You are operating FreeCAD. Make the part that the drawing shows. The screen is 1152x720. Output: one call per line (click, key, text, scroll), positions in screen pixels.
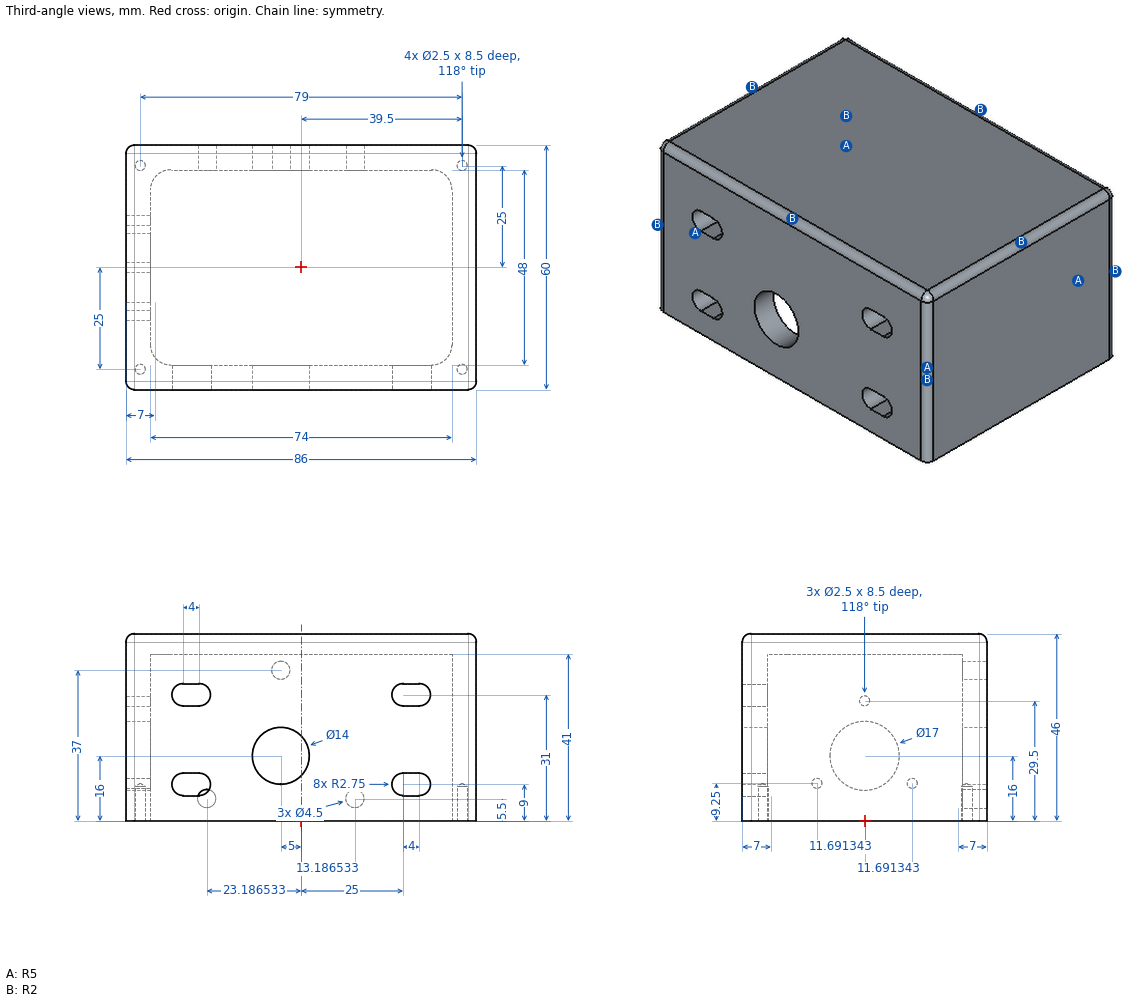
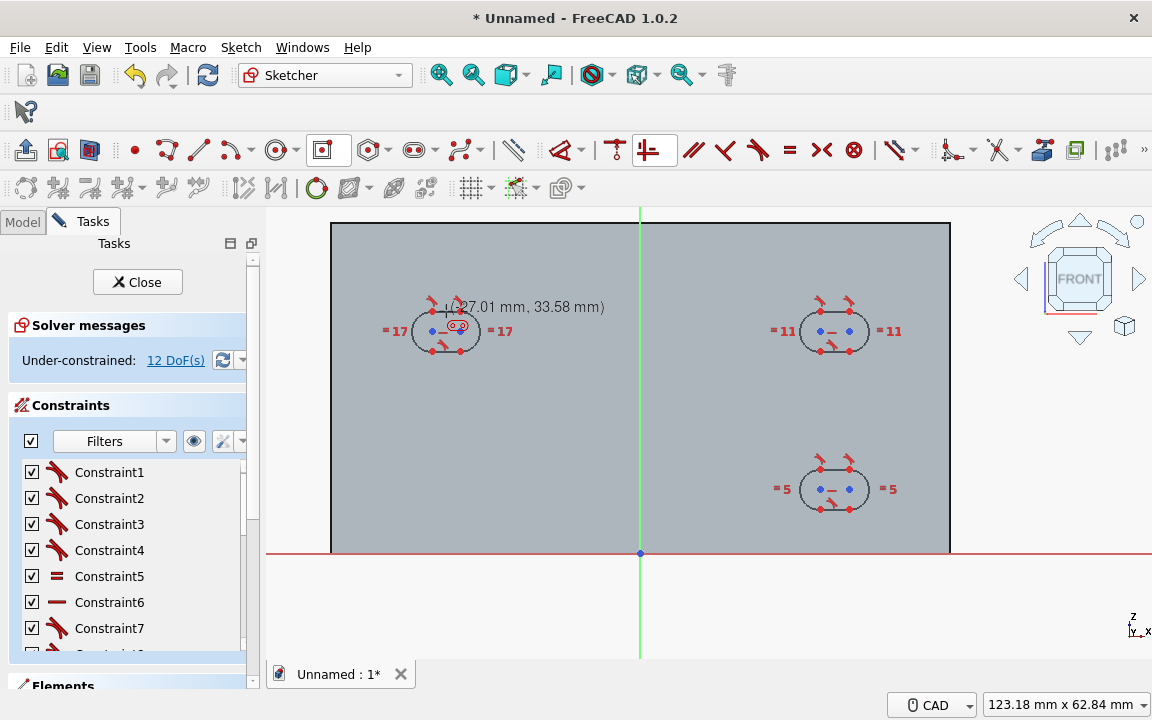
click(432, 489)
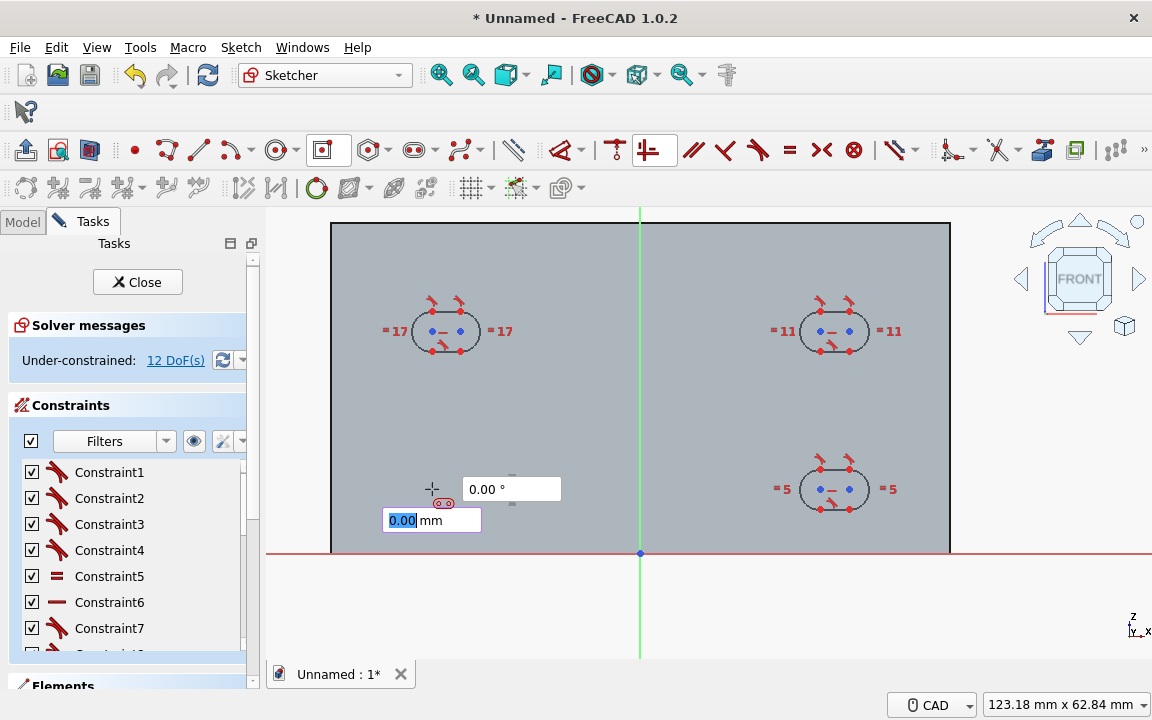
click(460, 489)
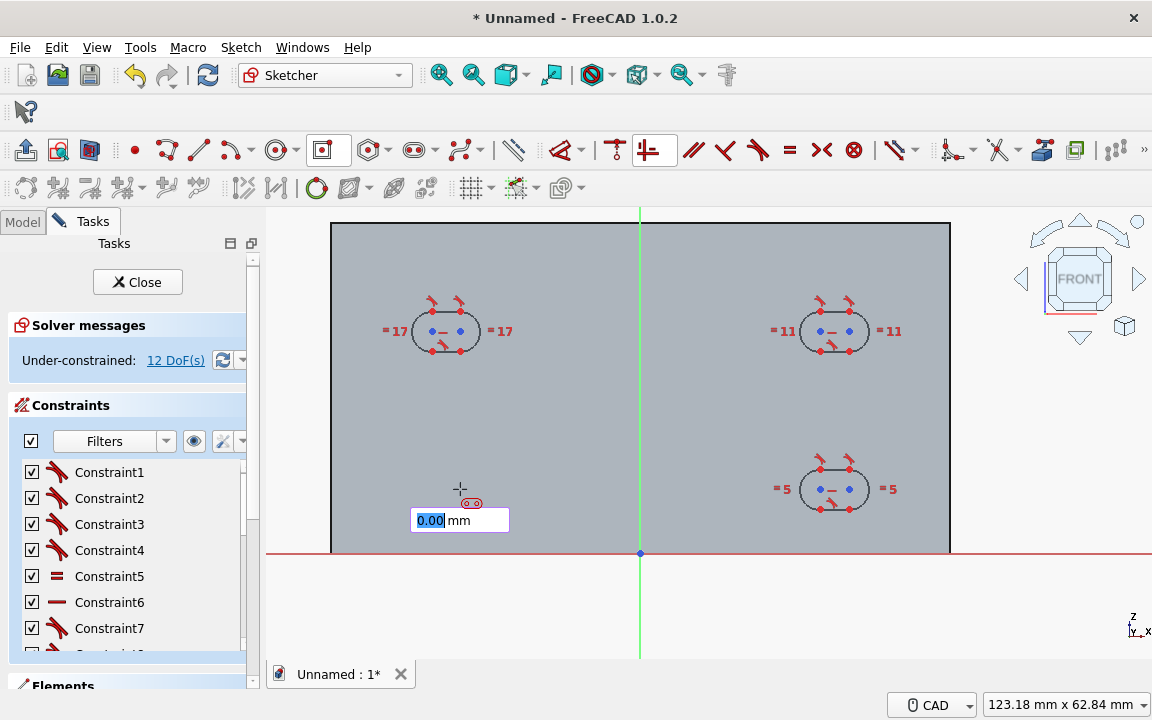
click(446, 469)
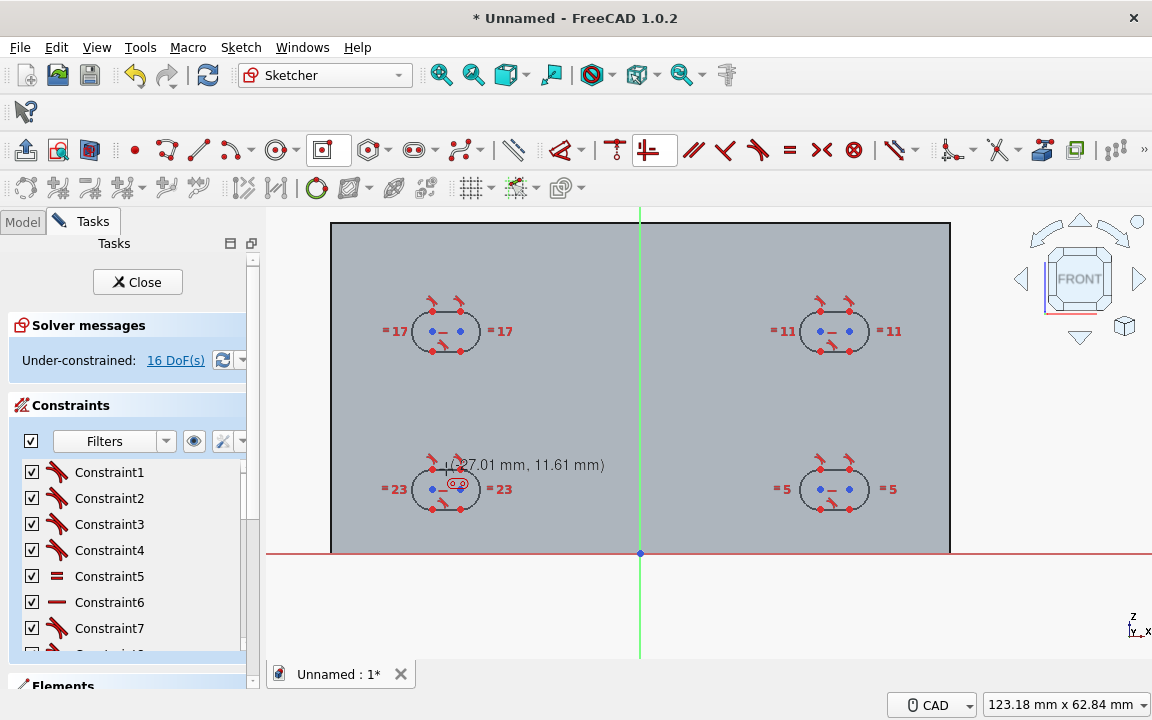
click(276, 150)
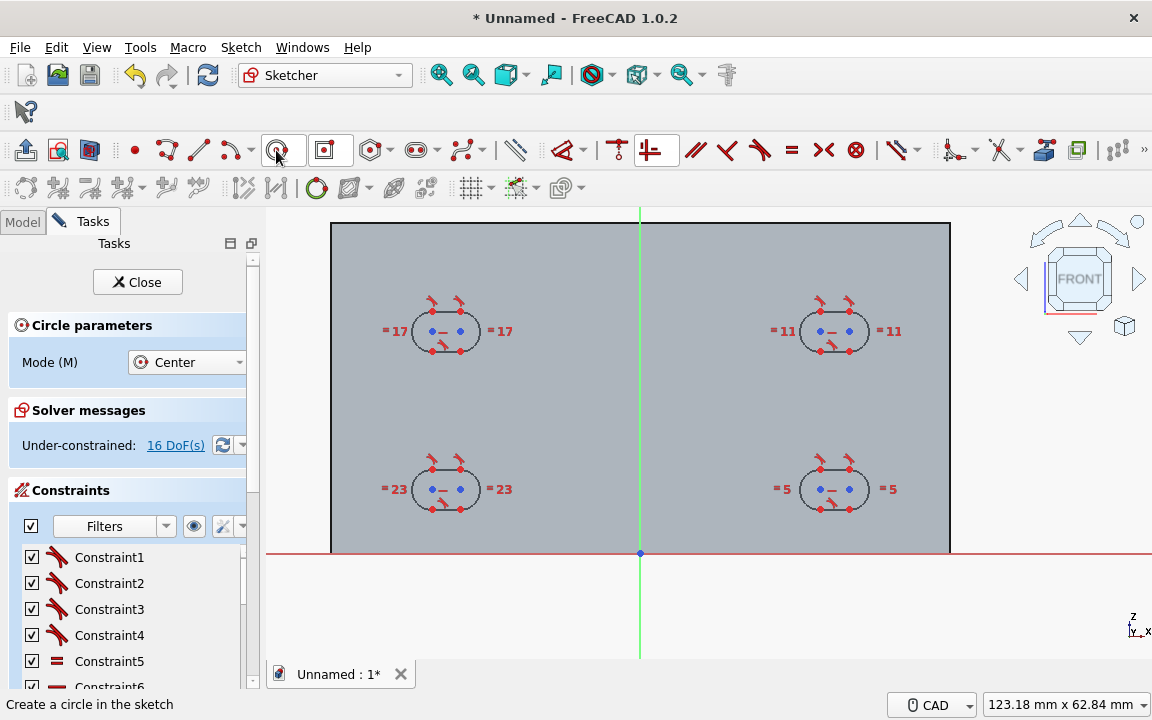
click(604, 438)
click(569, 403)
key(Escape)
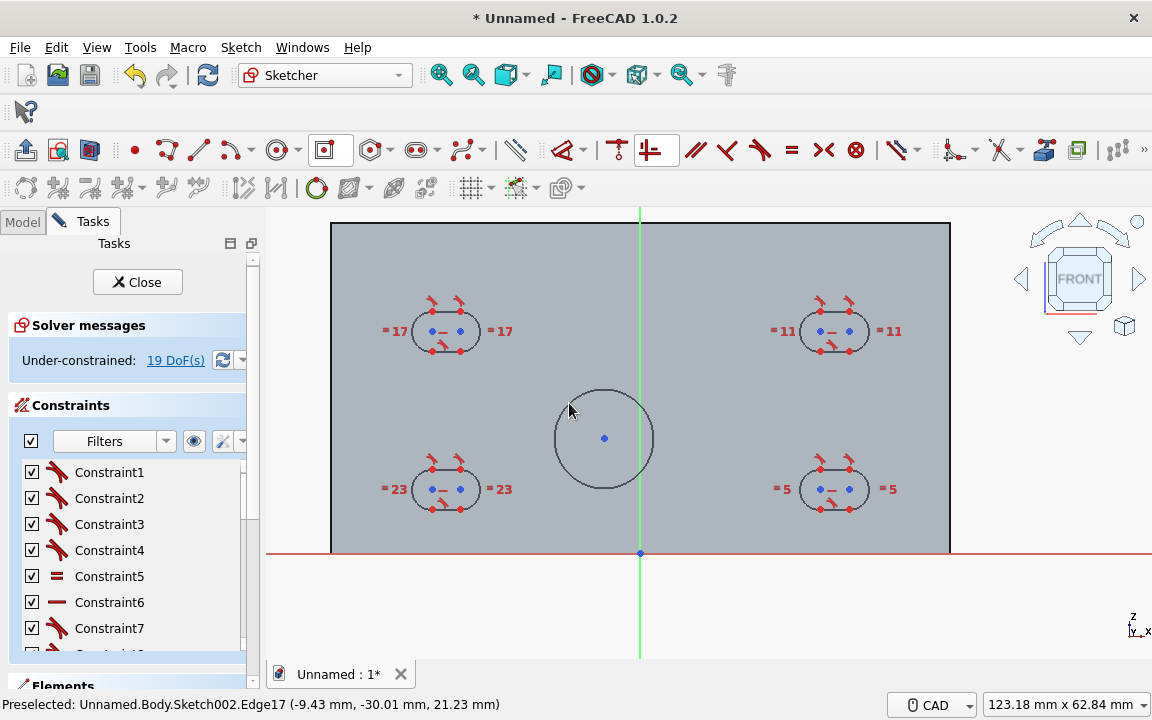
click(804, 478)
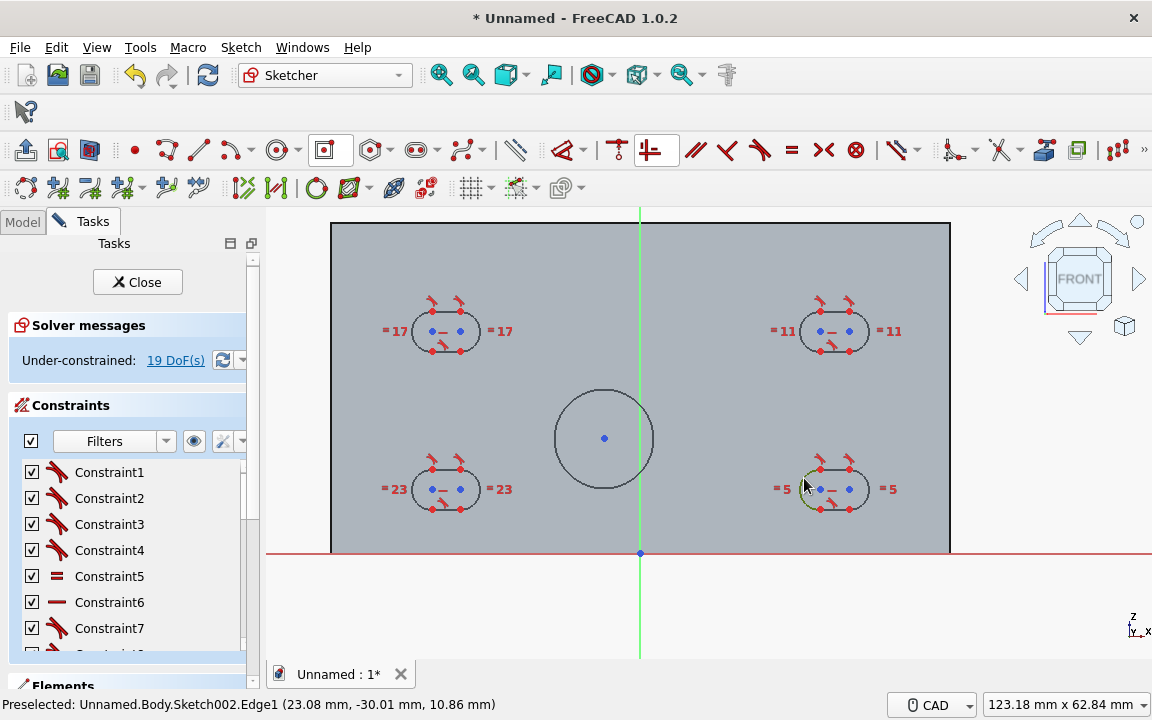
click(804, 320)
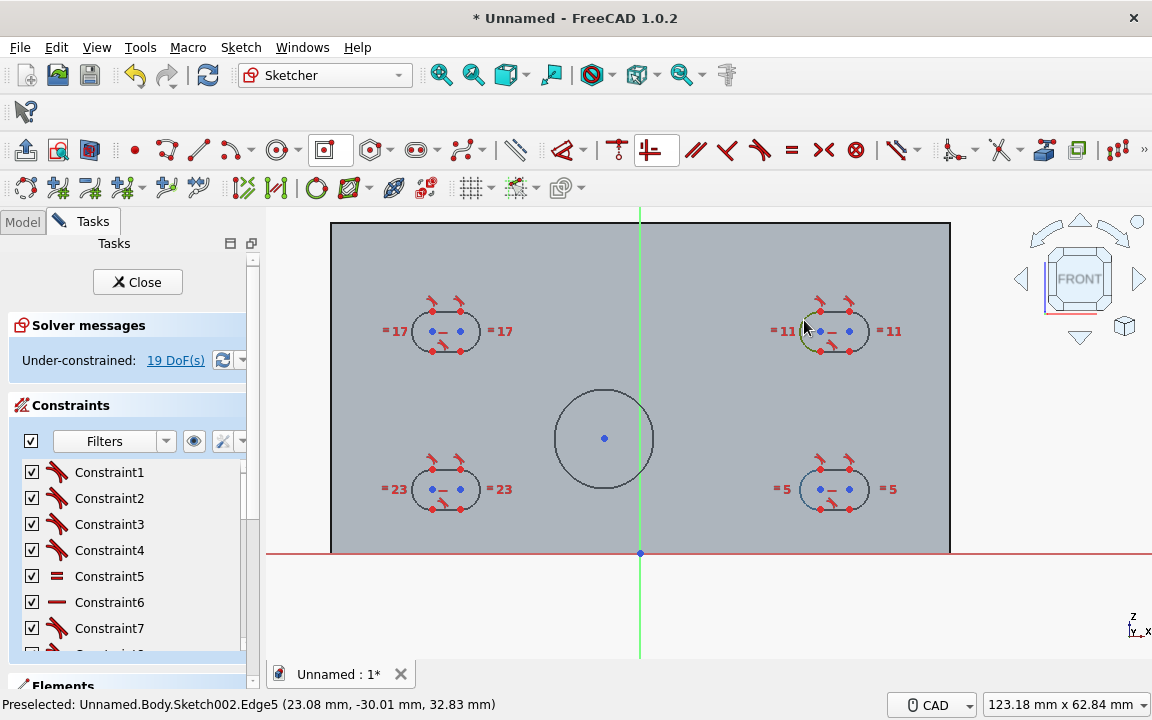
click(416, 320)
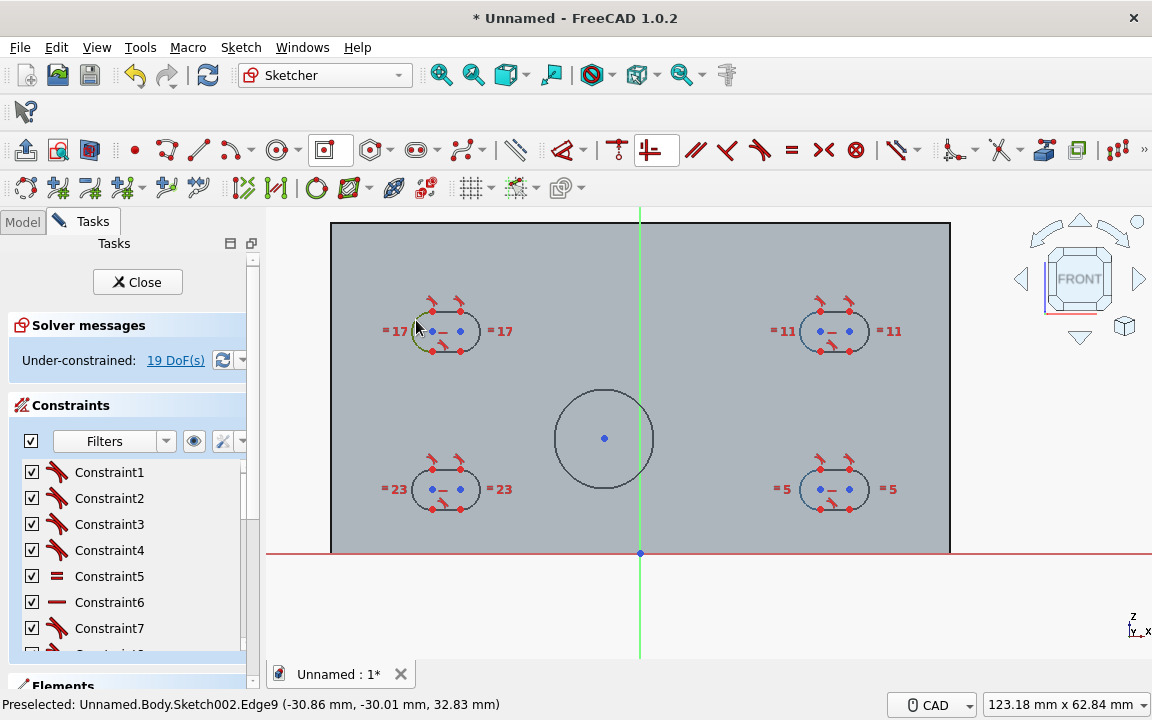
click(416, 478)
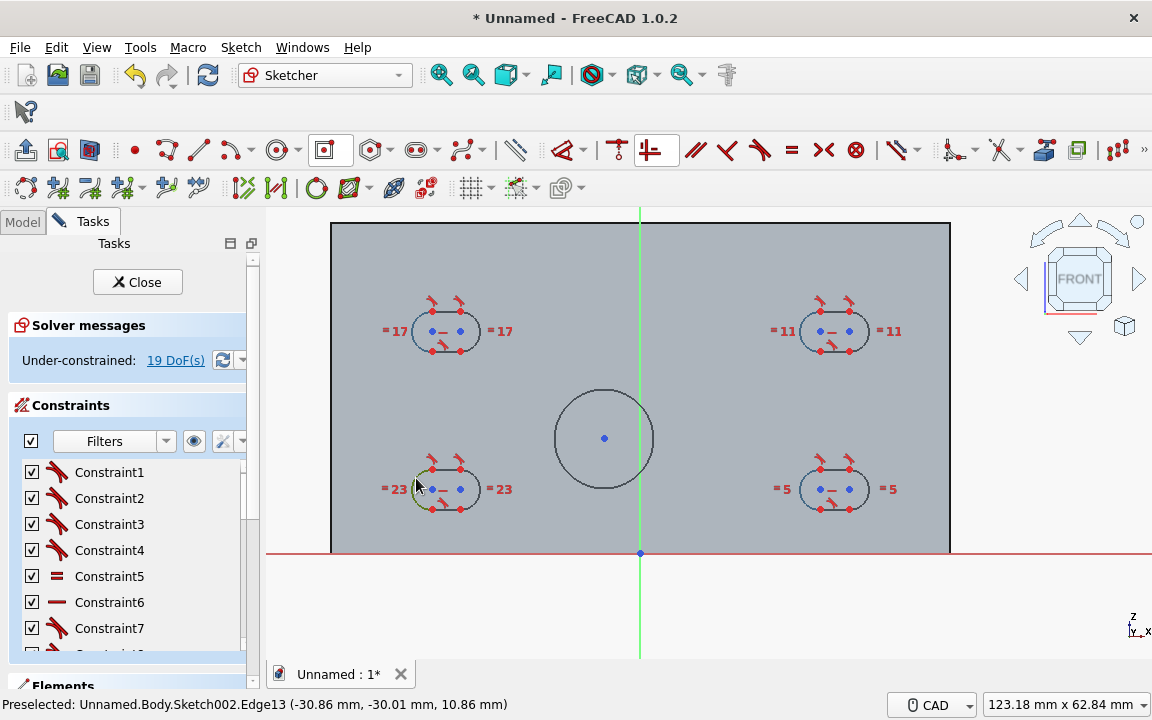
key(e)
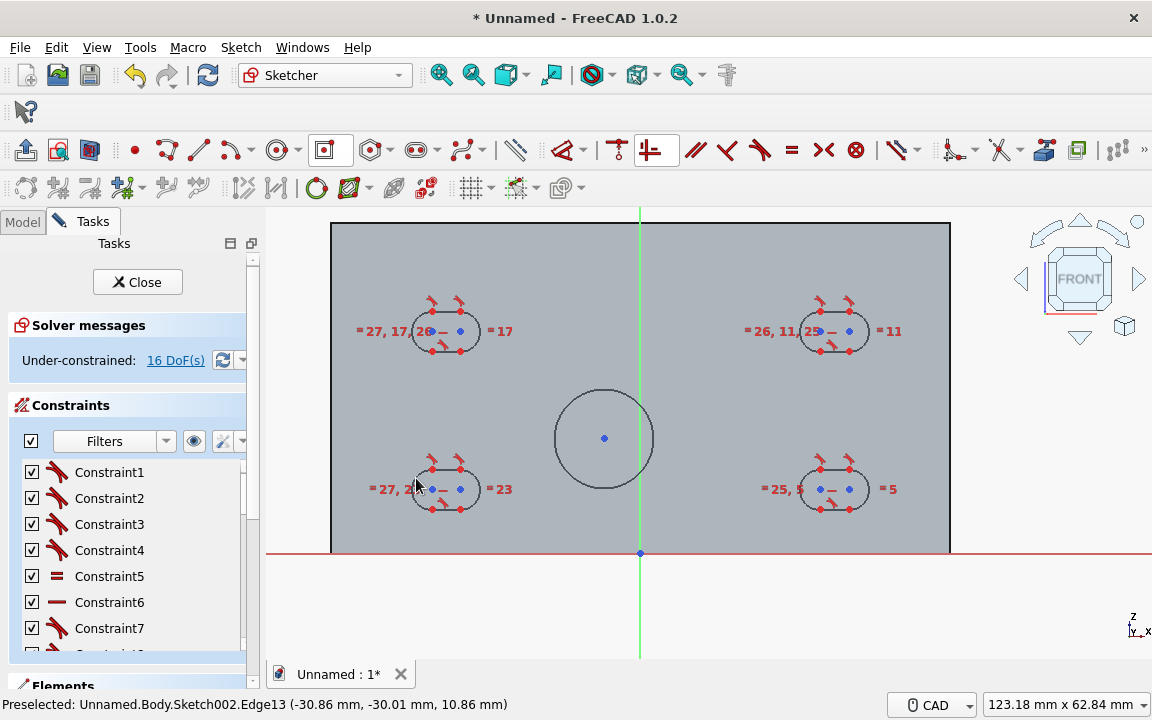
click(849, 332)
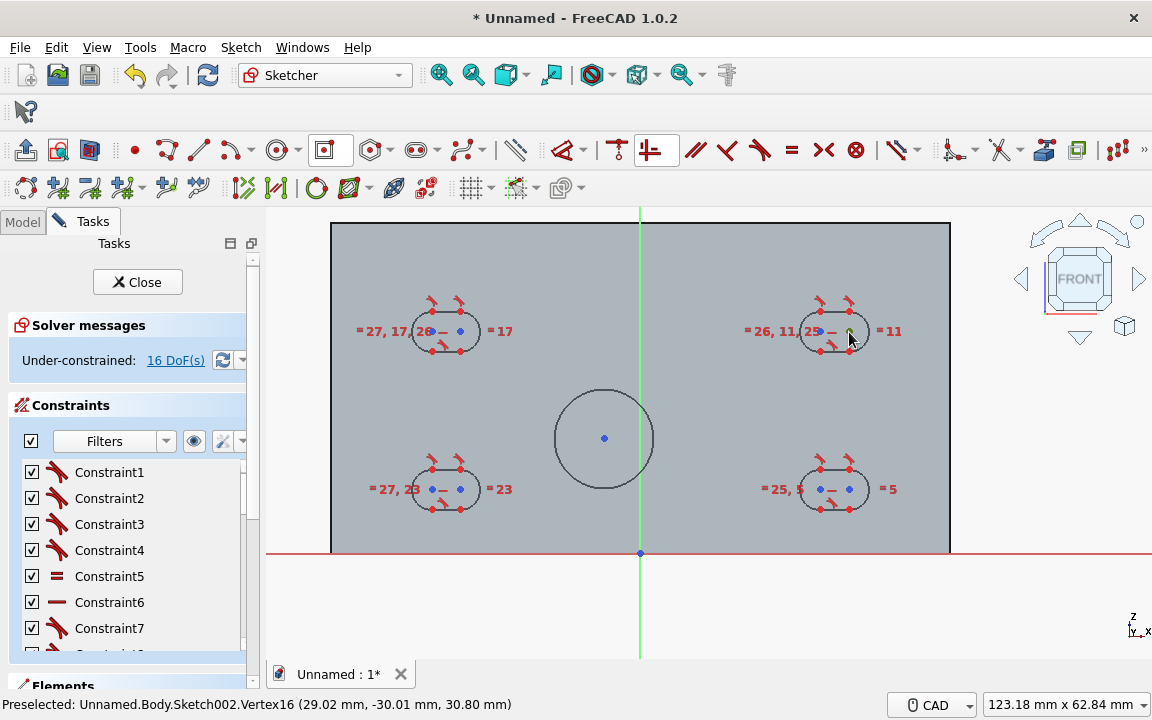
click(432, 332)